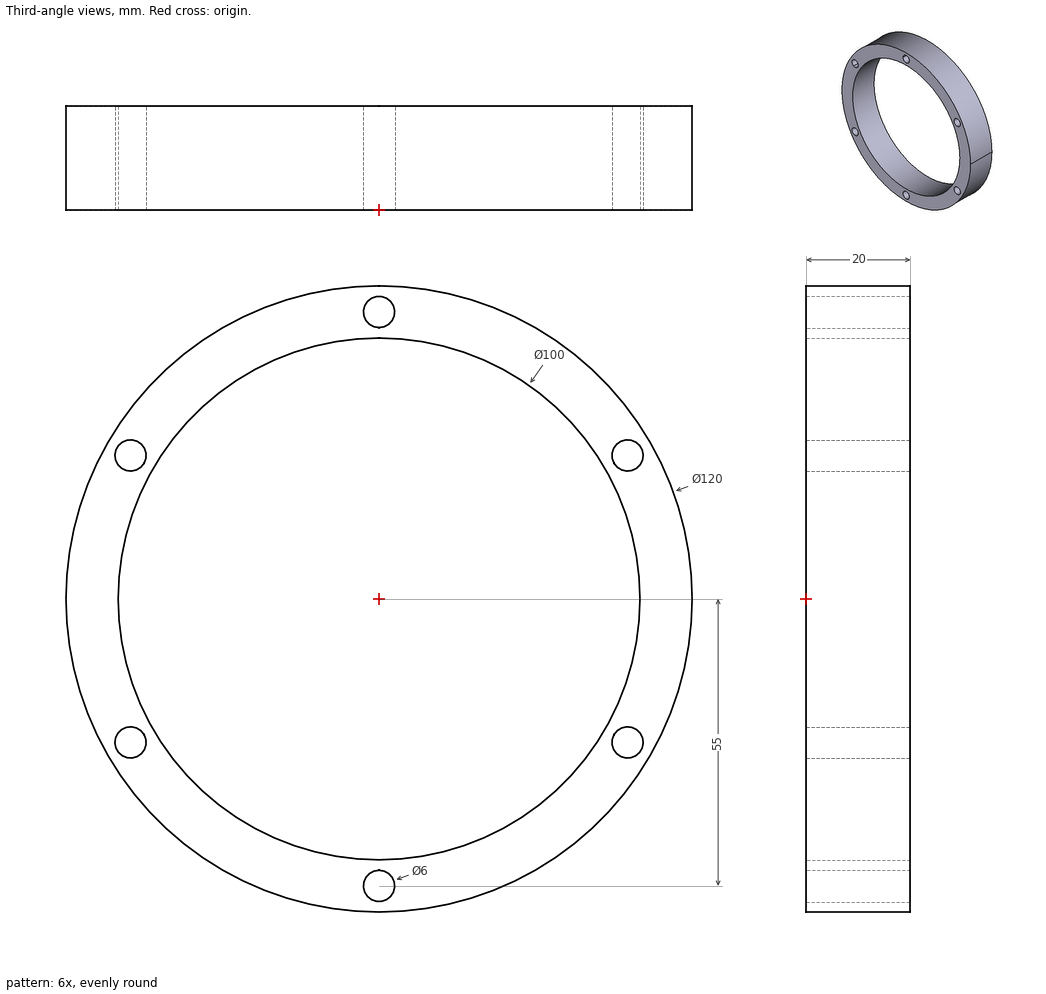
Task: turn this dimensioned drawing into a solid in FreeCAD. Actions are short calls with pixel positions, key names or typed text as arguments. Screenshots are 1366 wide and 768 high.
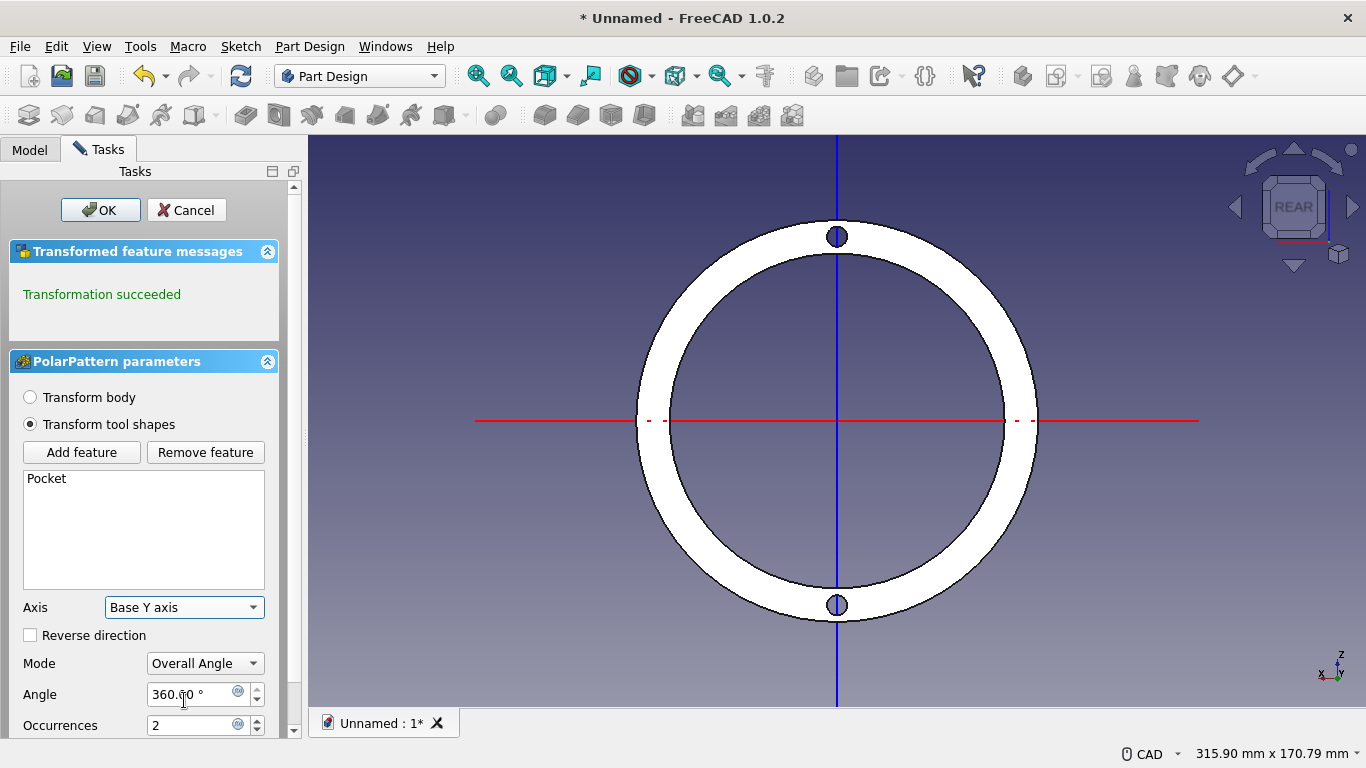
triple_click(199, 726)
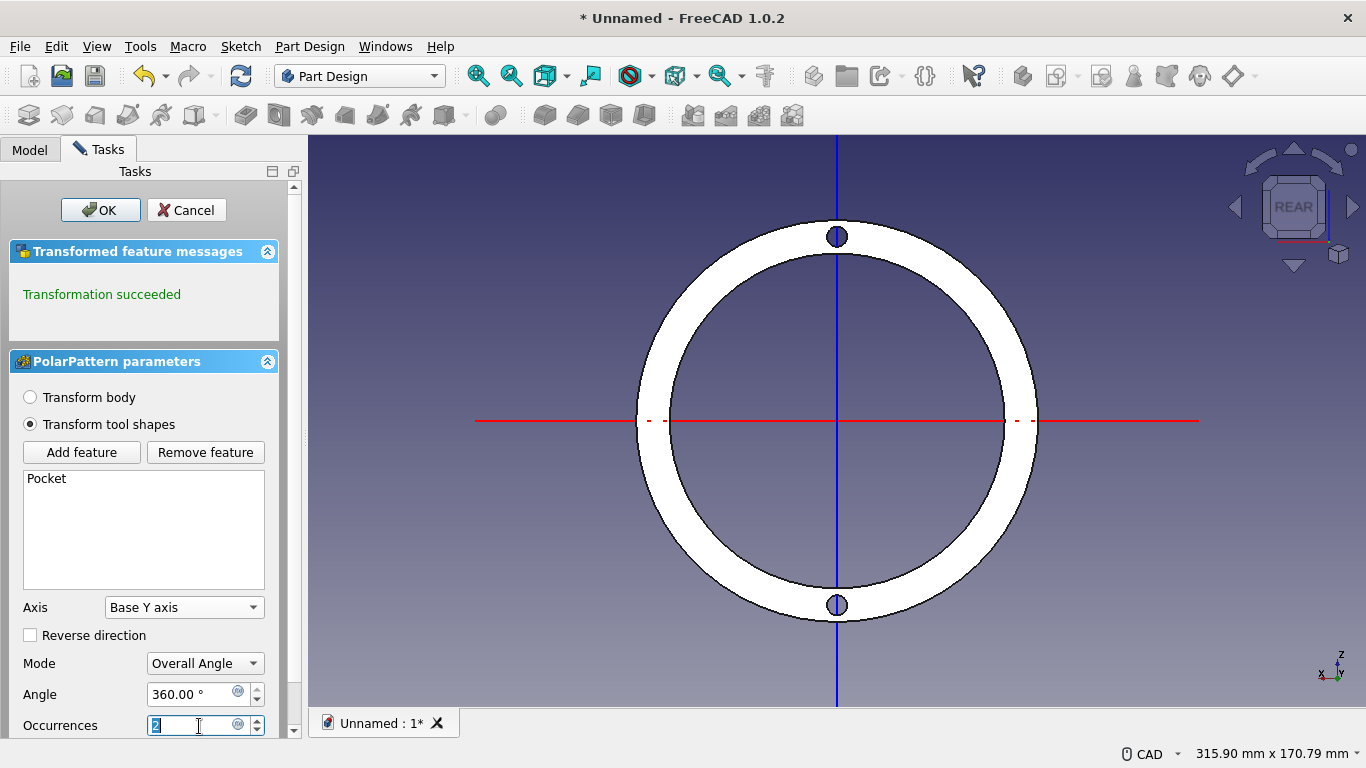
text(6)
key(Tab)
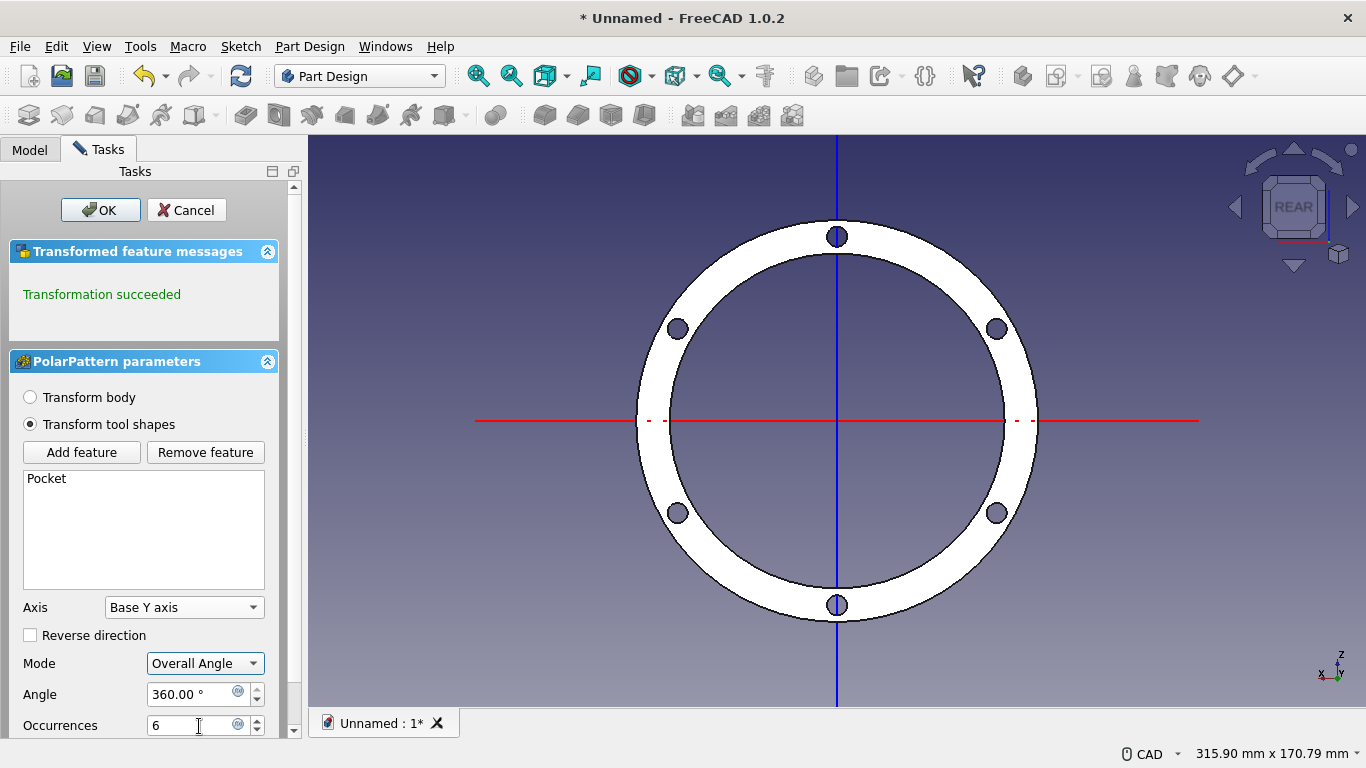
click(101, 210)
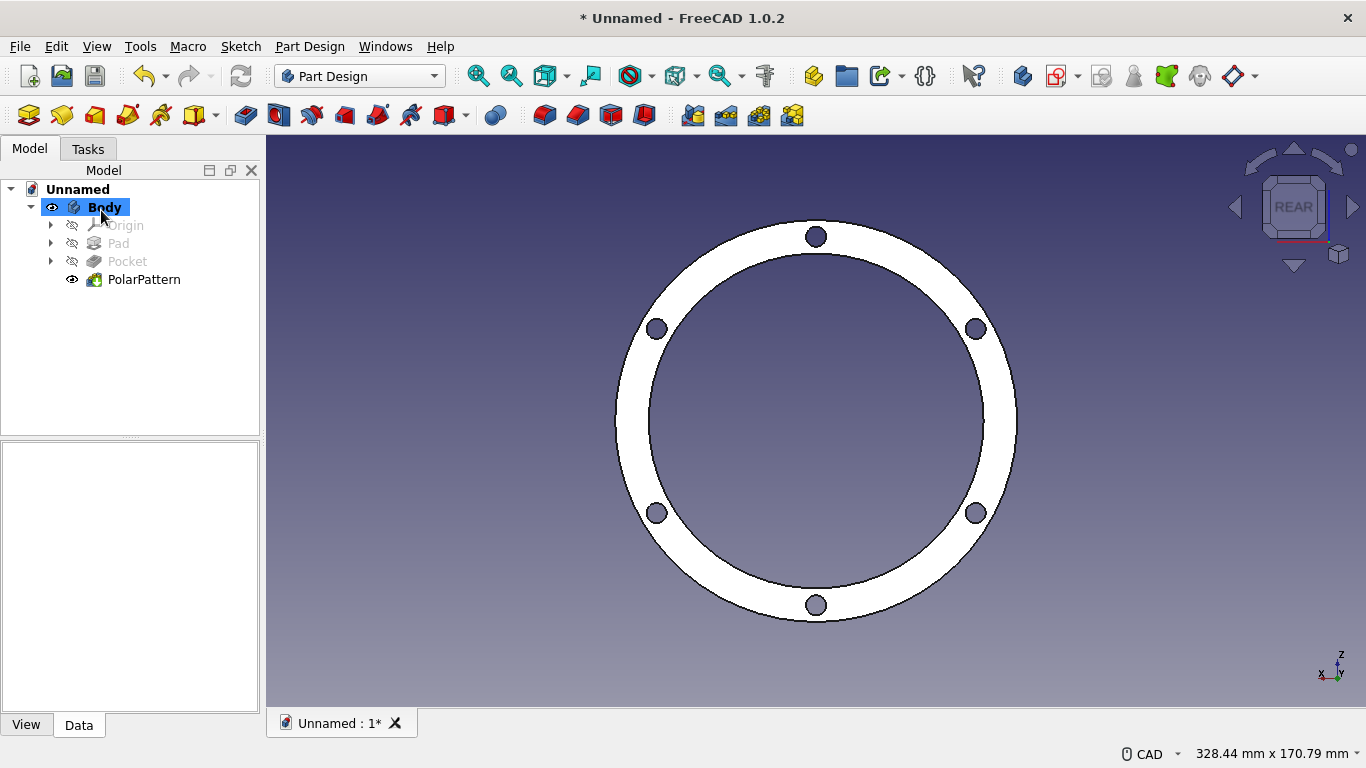
key(0)